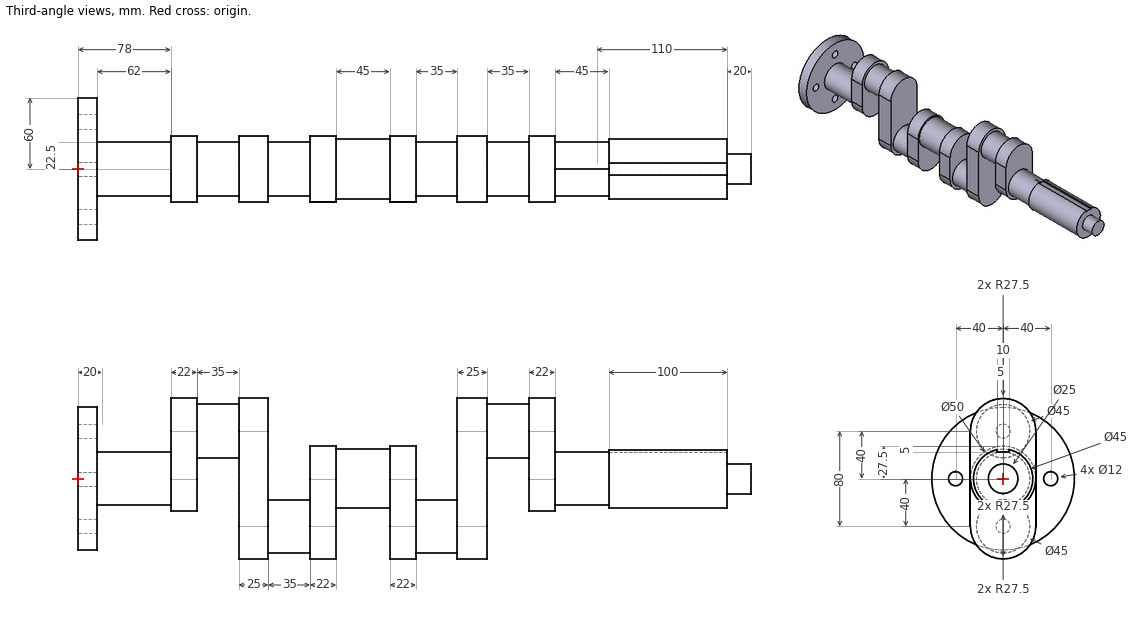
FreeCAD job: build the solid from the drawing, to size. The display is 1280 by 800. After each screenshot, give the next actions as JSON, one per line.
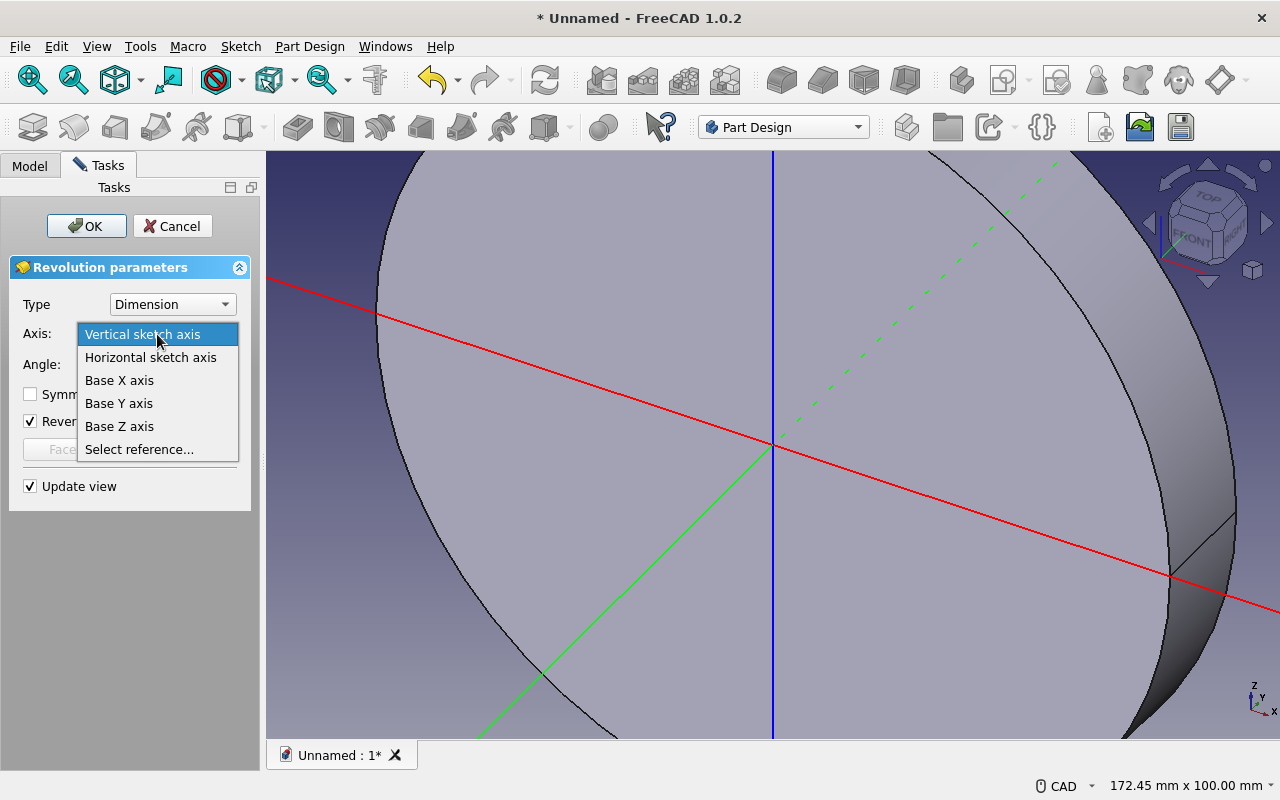
{"action": "left_click", "coordinate": [156, 358]}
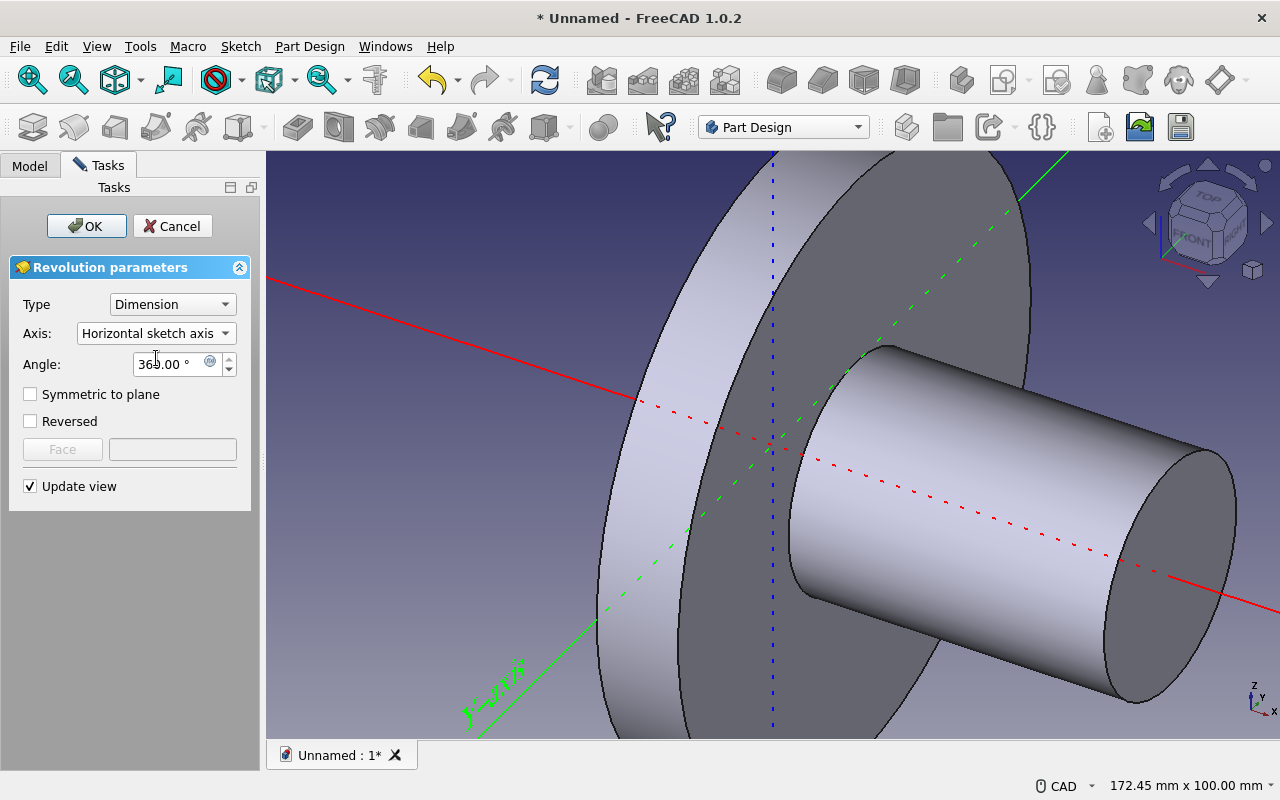
{"action": "left_click", "coordinate": [87, 226]}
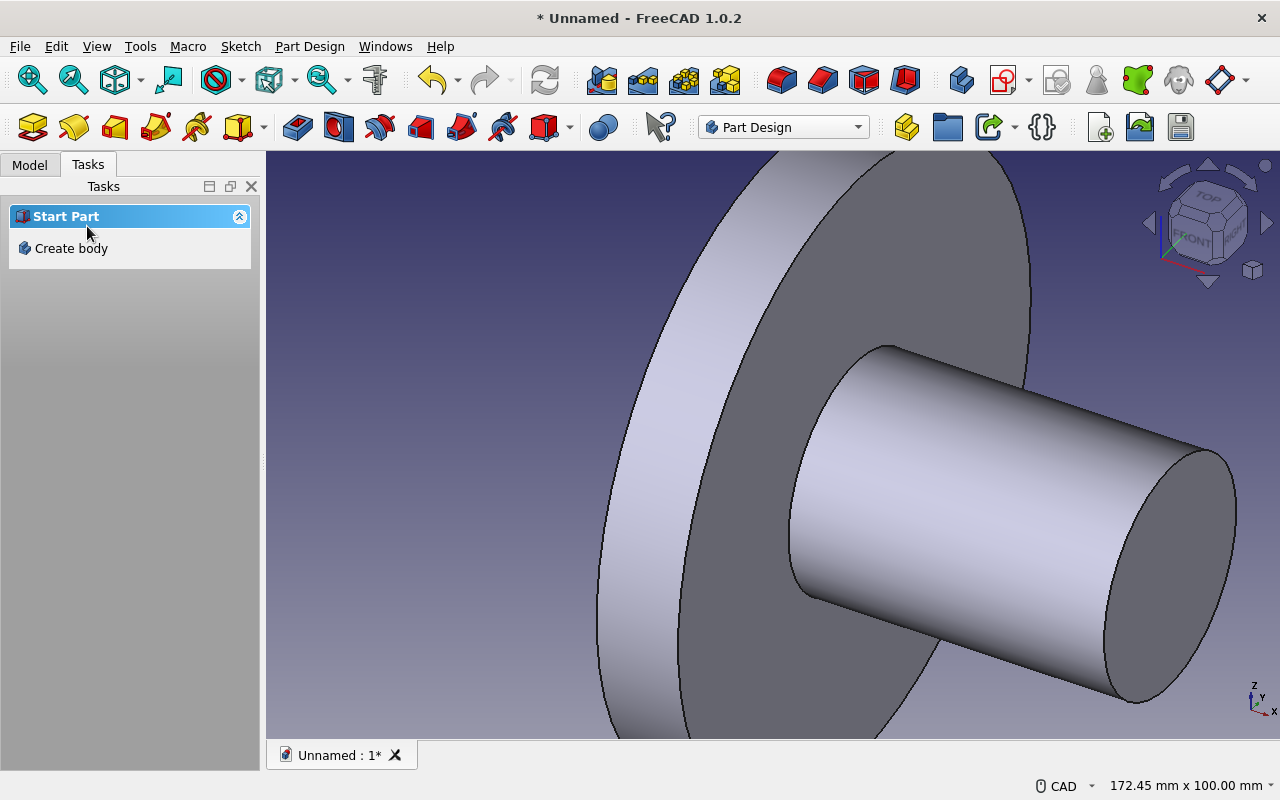
{"action": "left_click", "coordinate": [33, 80]}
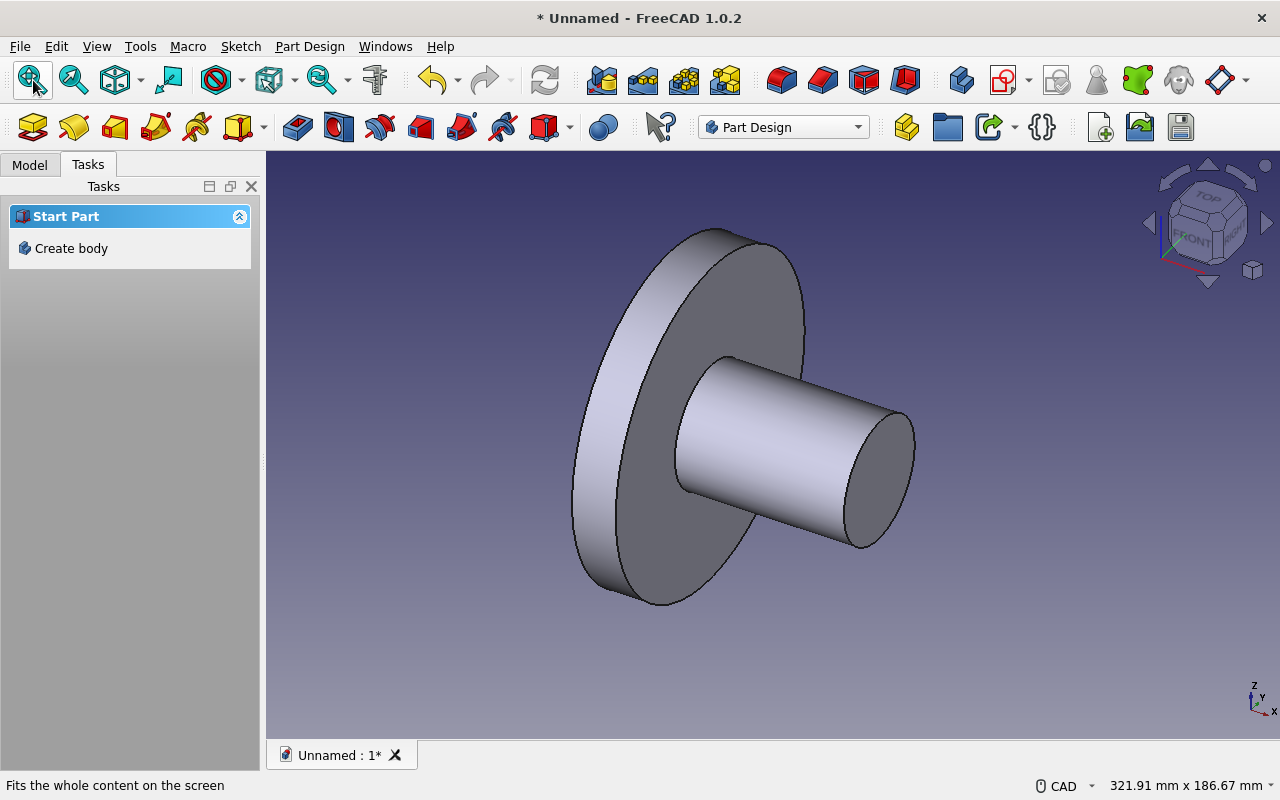
{"action": "left_click", "coordinate": [879, 479]}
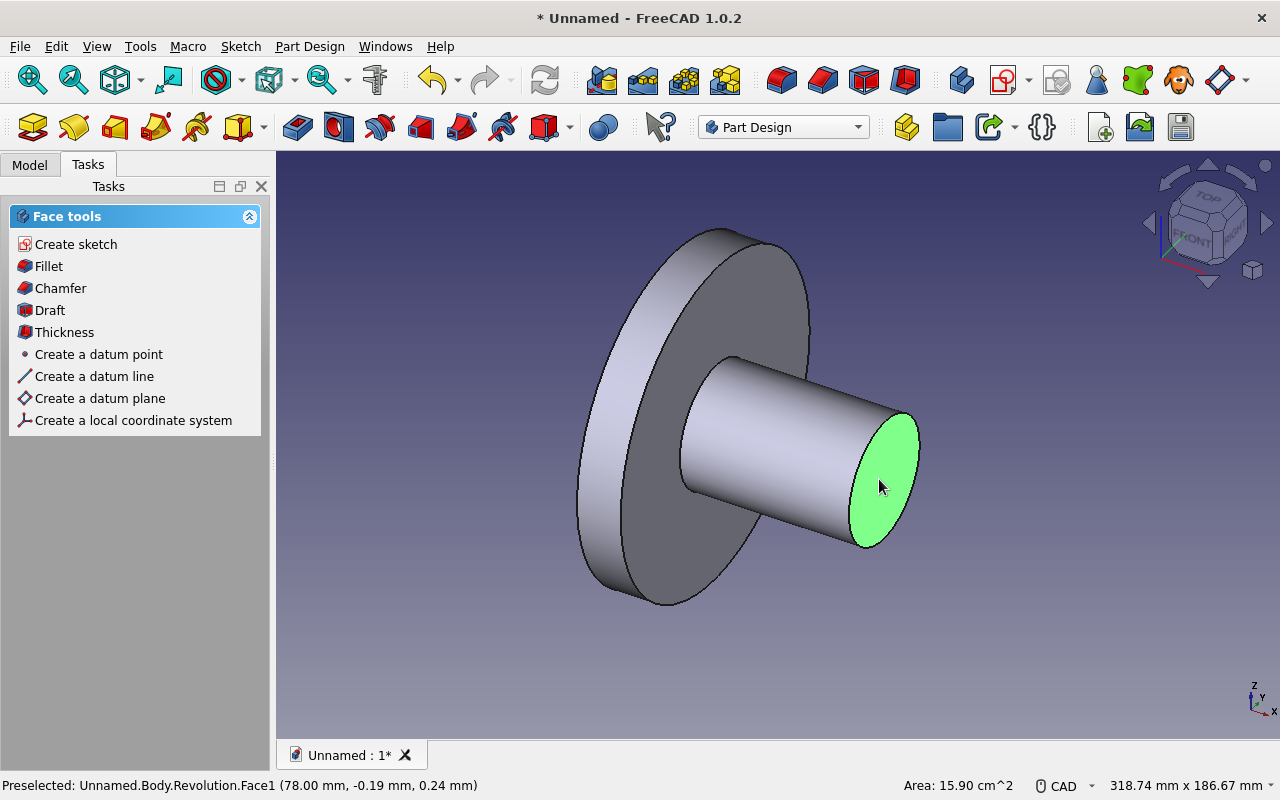
{"action": "left_click", "coordinate": [1002, 80]}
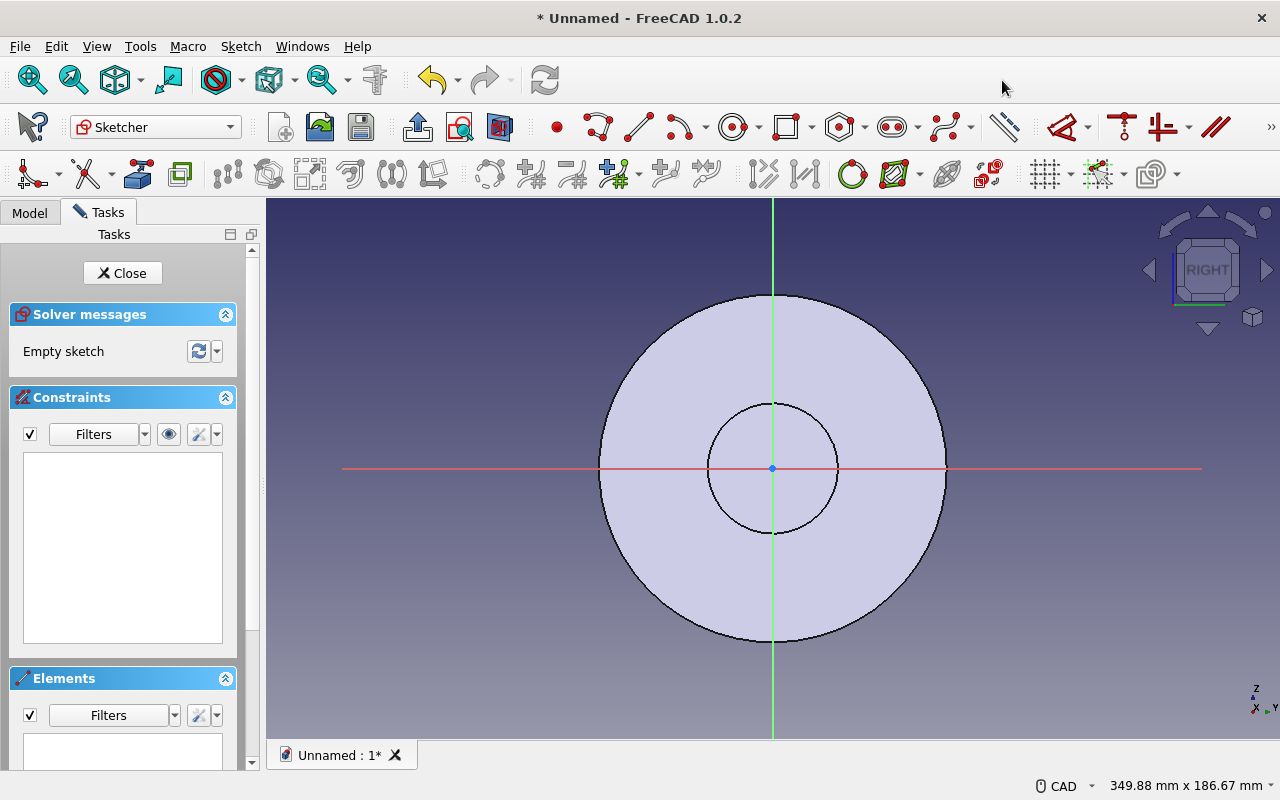
{"action": "left_click", "coordinate": [892, 128]}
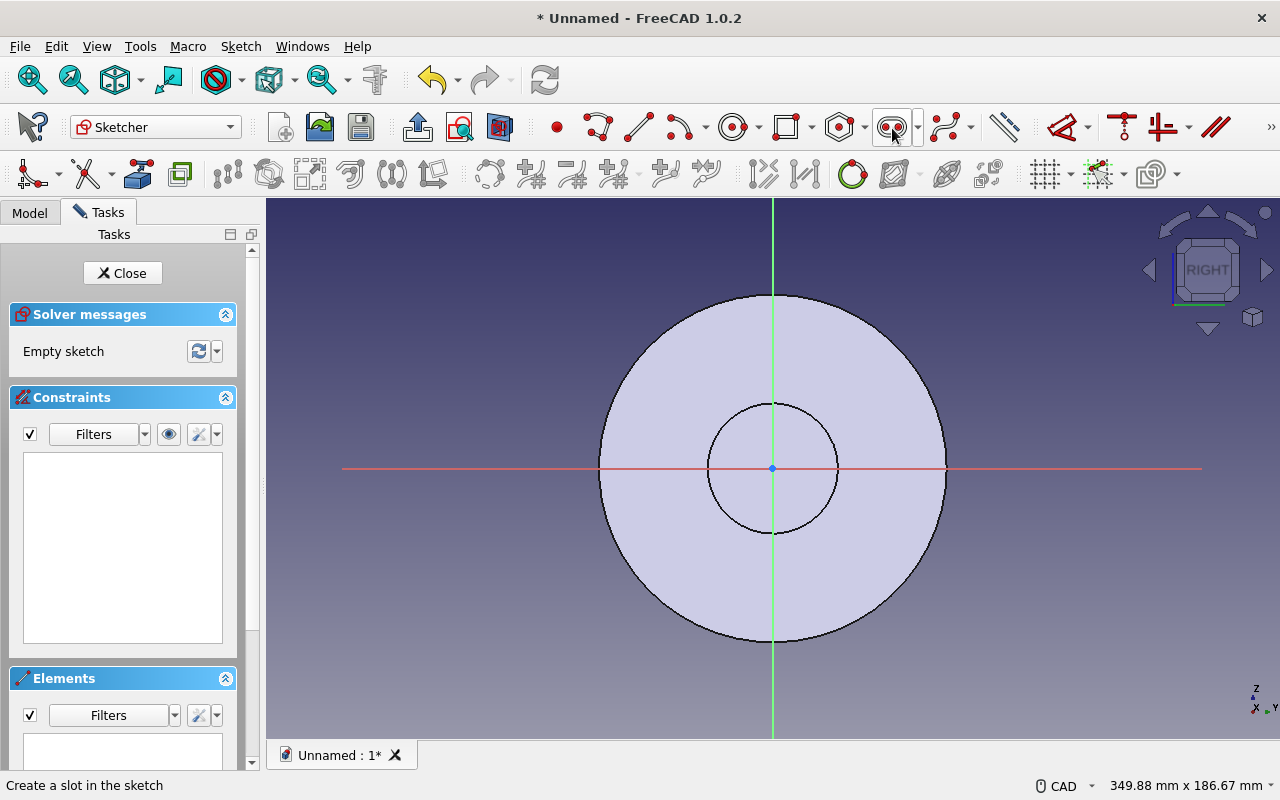
{"action": "left_click", "coordinate": [773, 468]}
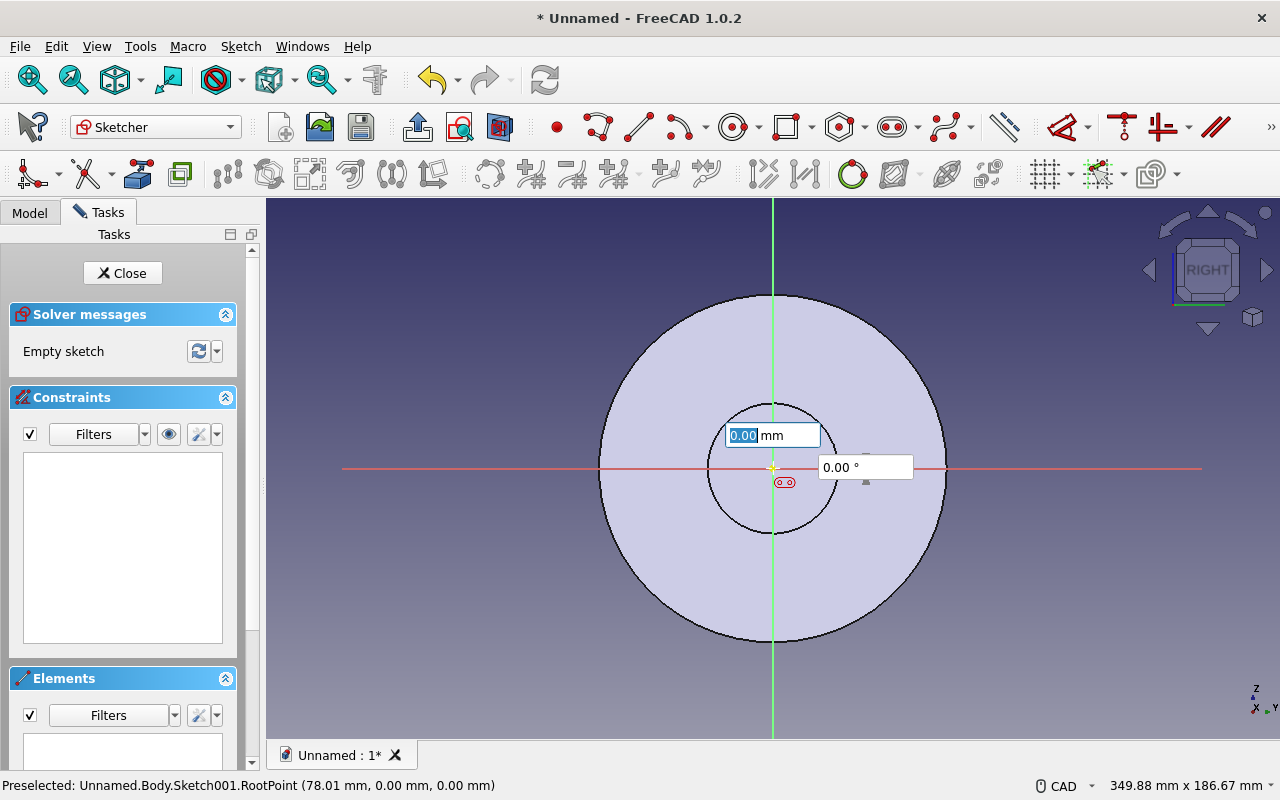
{"action": "left_click", "coordinate": [782, 353]}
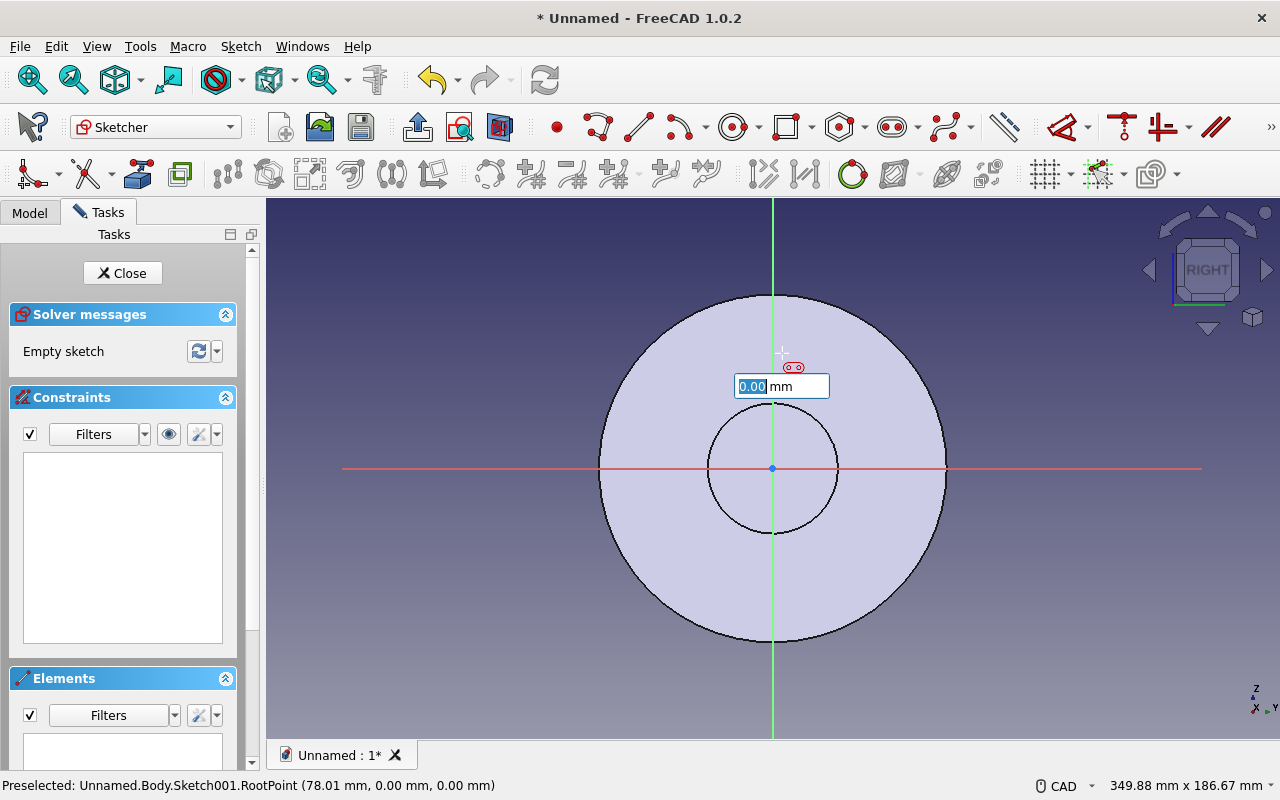
{"action": "left_click", "coordinate": [693, 411]}
{"action": "key", "text": "Escape"}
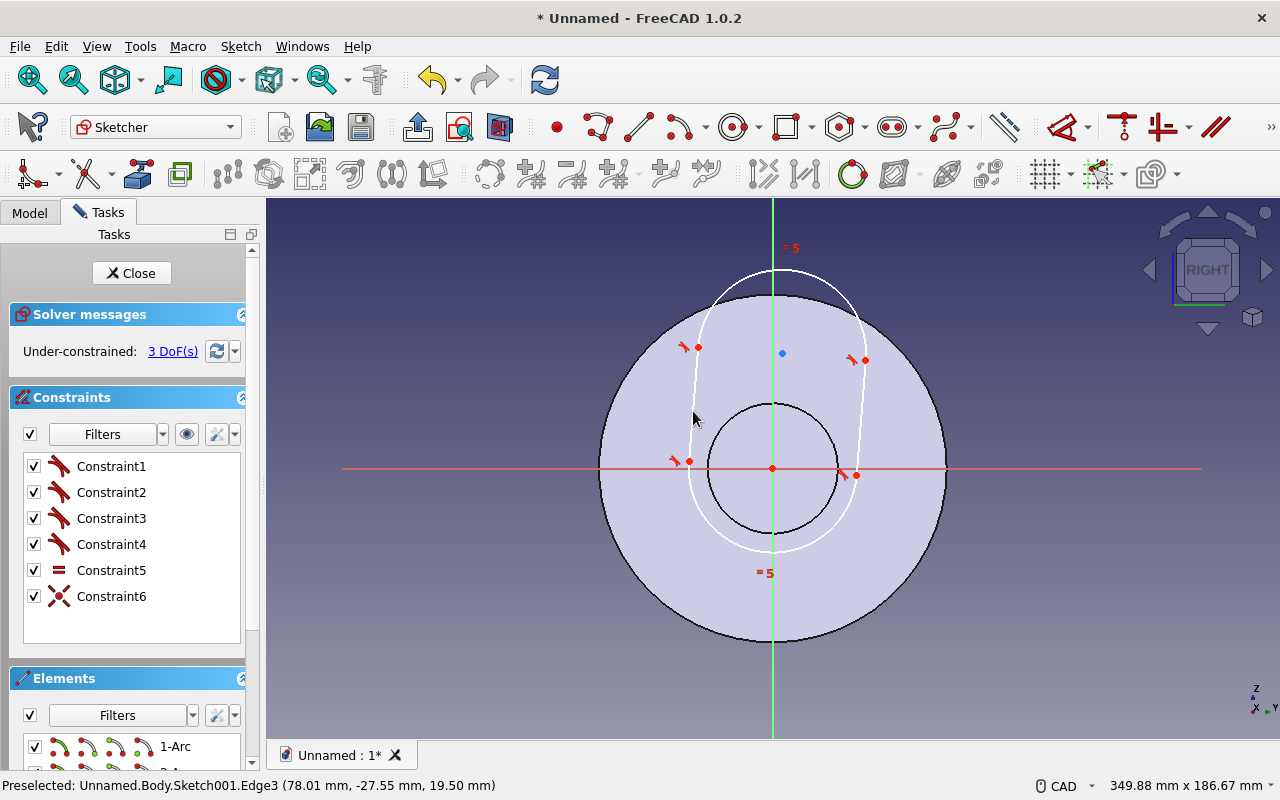
{"action": "left_click", "coordinate": [692, 427]}